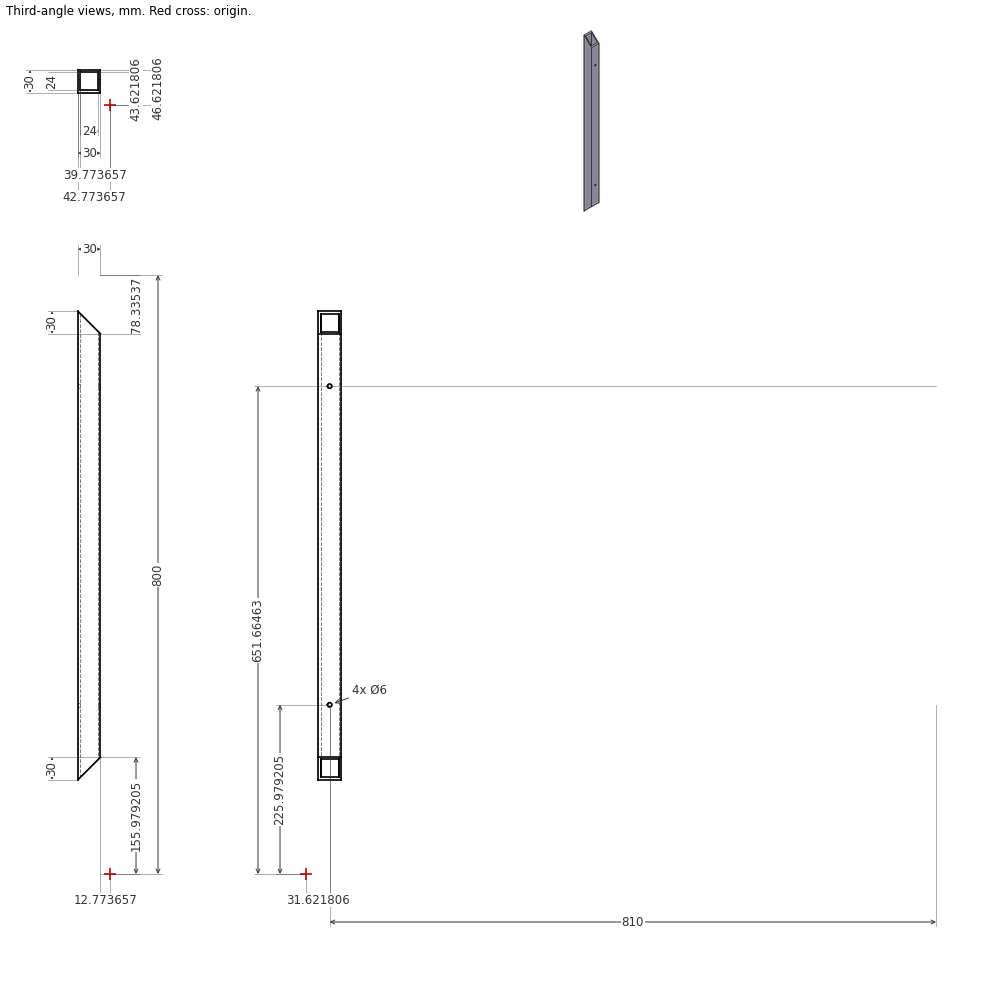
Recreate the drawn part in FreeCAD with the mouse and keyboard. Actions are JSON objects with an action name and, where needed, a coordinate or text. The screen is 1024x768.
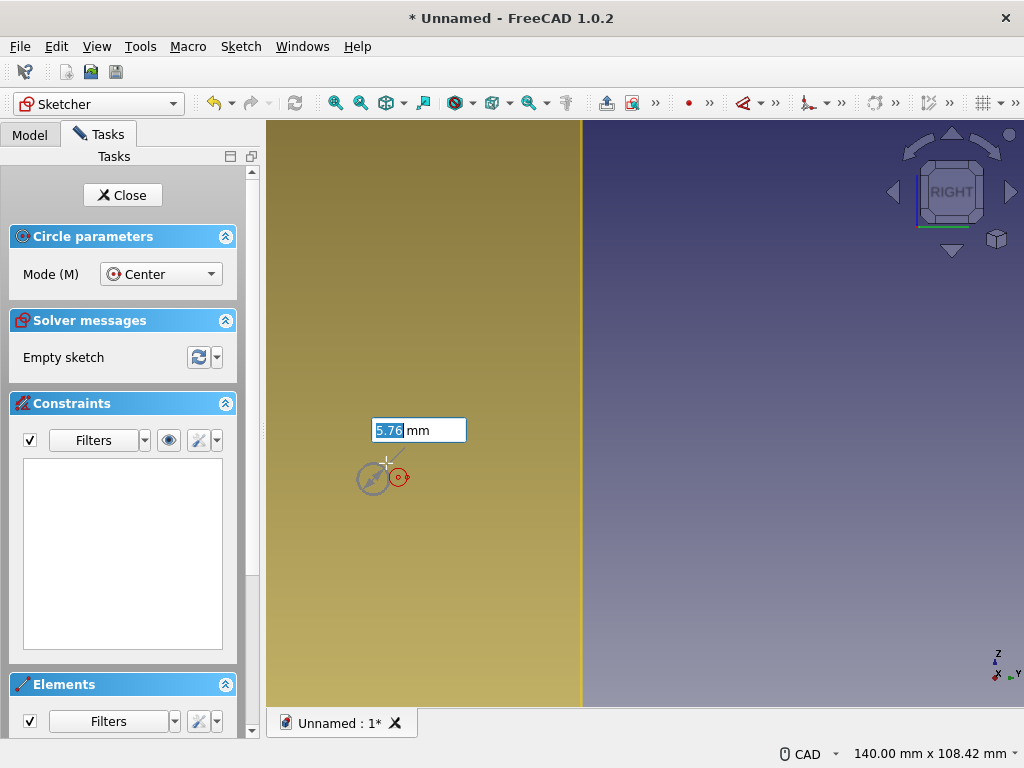
{"action": "left_click", "coordinate": [384, 454]}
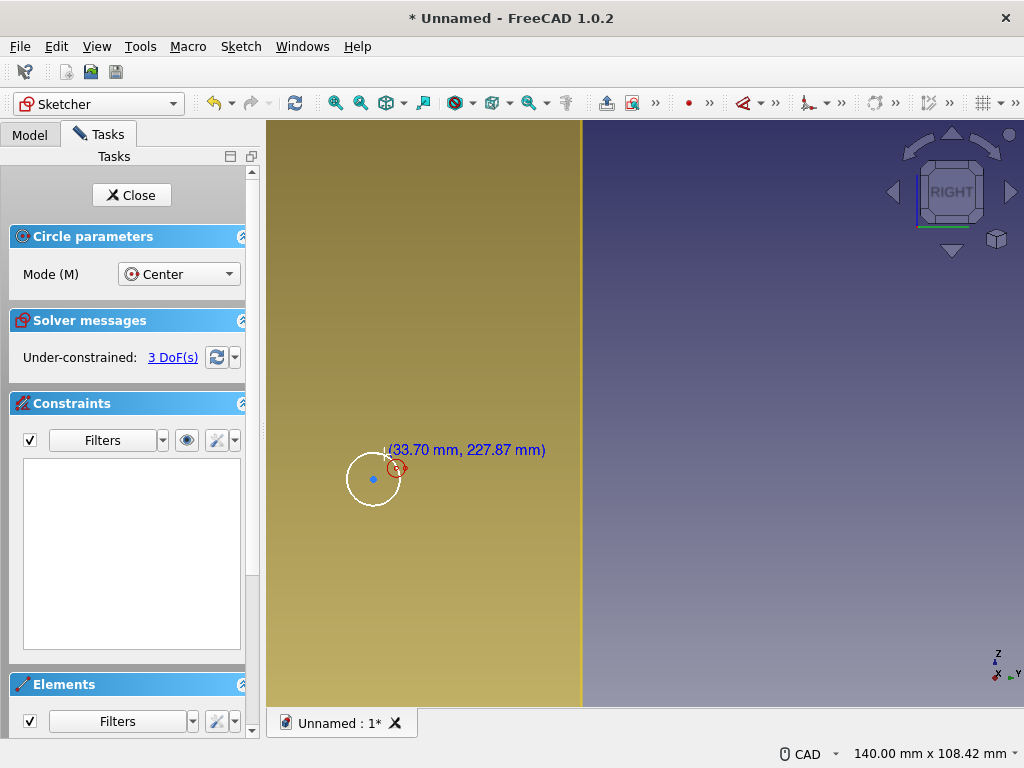
{"action": "scroll", "coordinate": [386, 463], "scroll_direction": "down", "scroll_amount": 12}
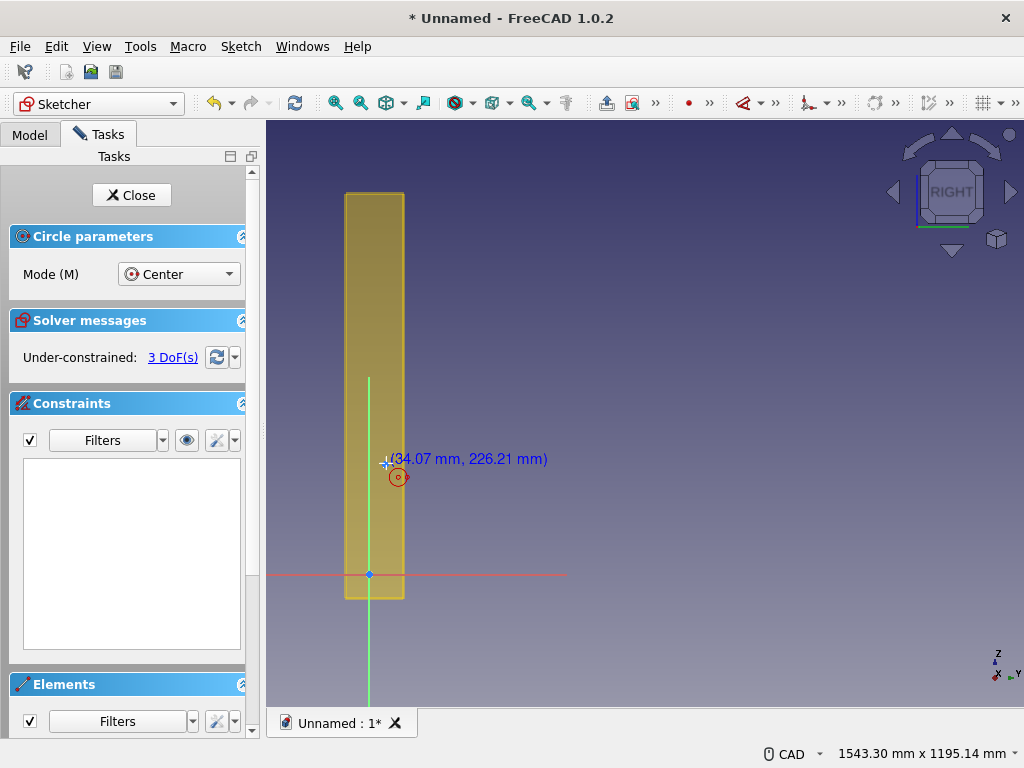
{"action": "scroll", "coordinate": [783, 464], "scroll_direction": "up", "scroll_amount": 14}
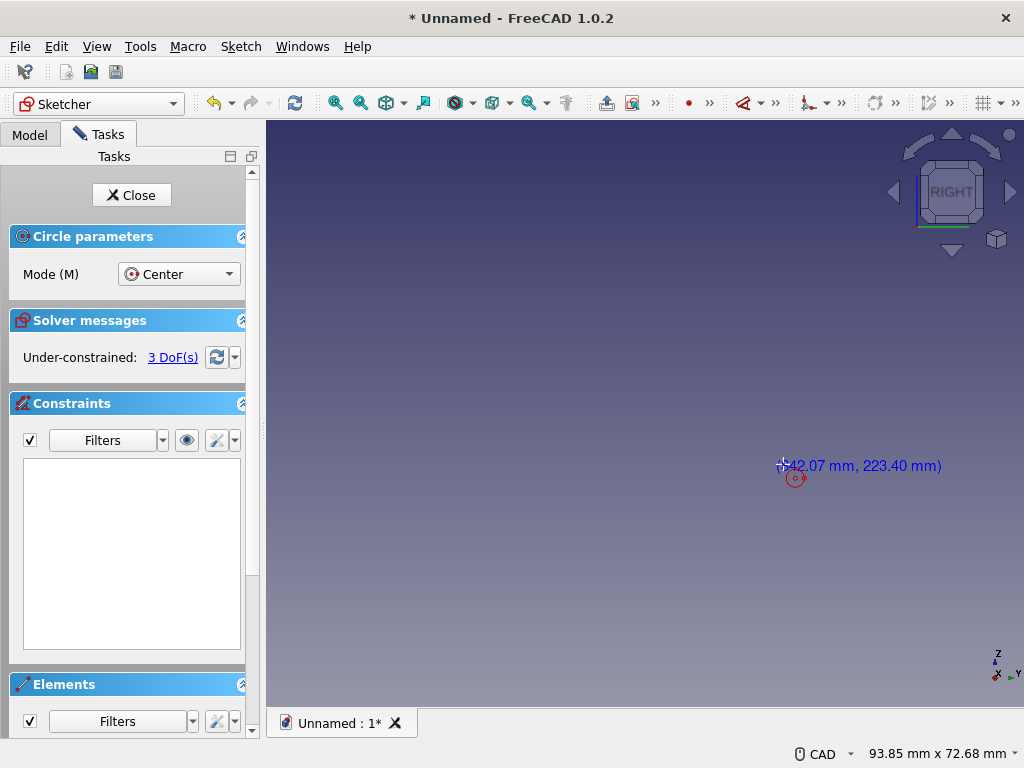
{"action": "scroll", "coordinate": [783, 464], "scroll_direction": "down", "scroll_amount": 14}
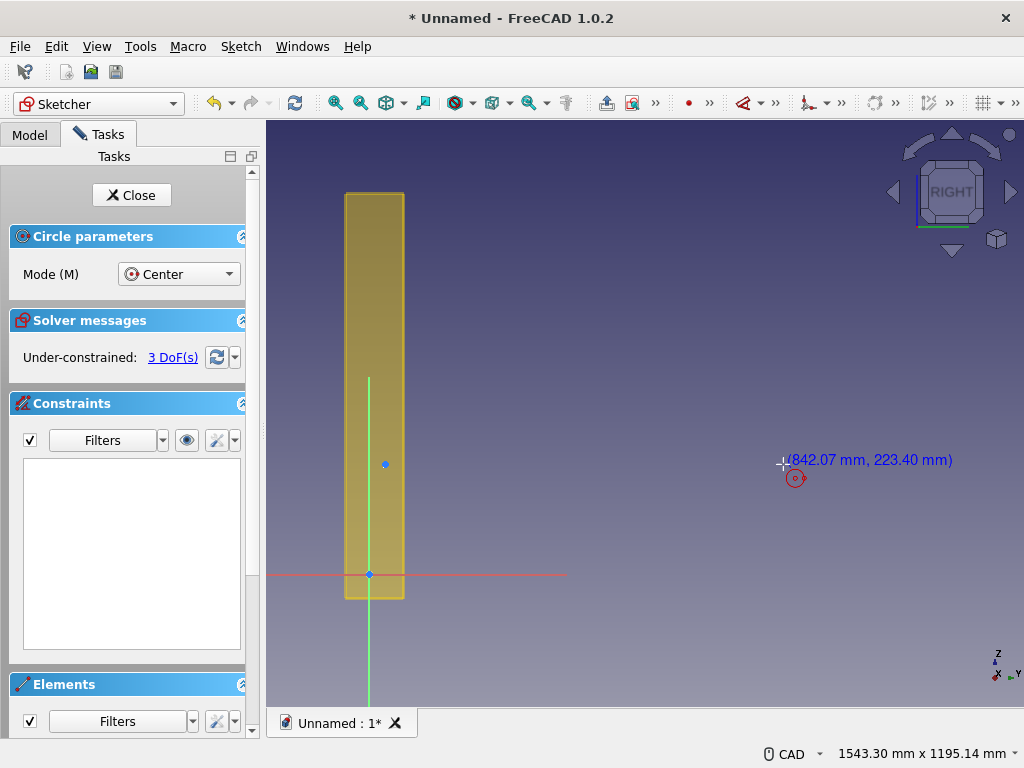
{"action": "left_click", "coordinate": [783, 464]}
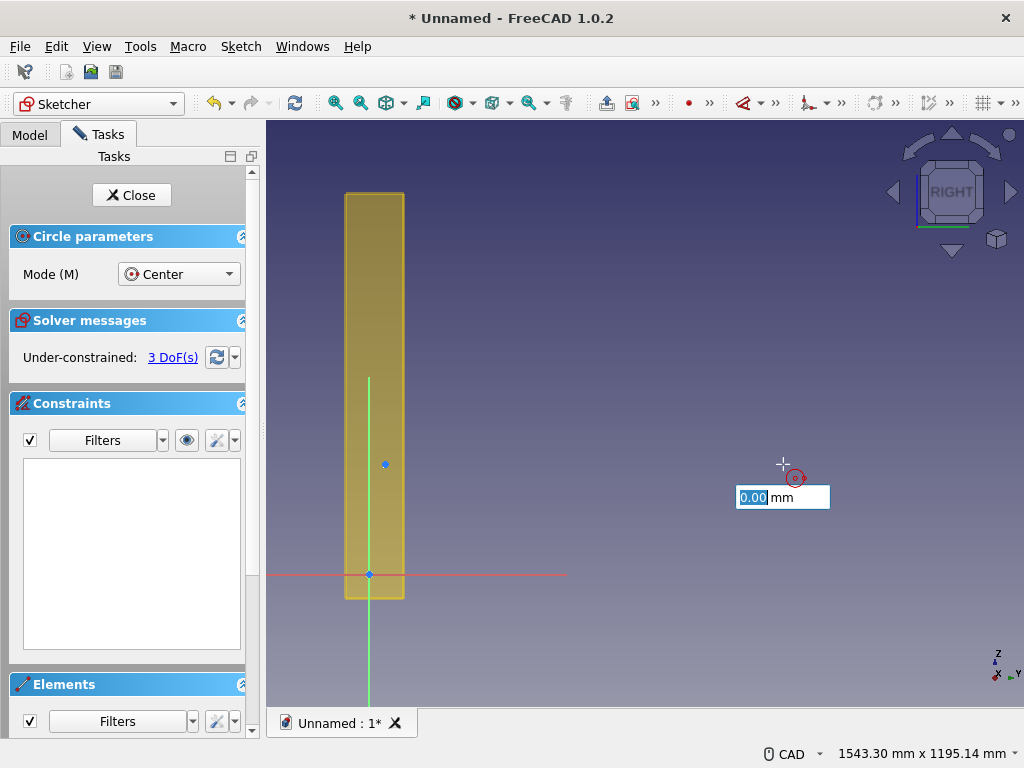
{"action": "scroll", "coordinate": [784, 463], "scroll_direction": "up", "scroll_amount": 12}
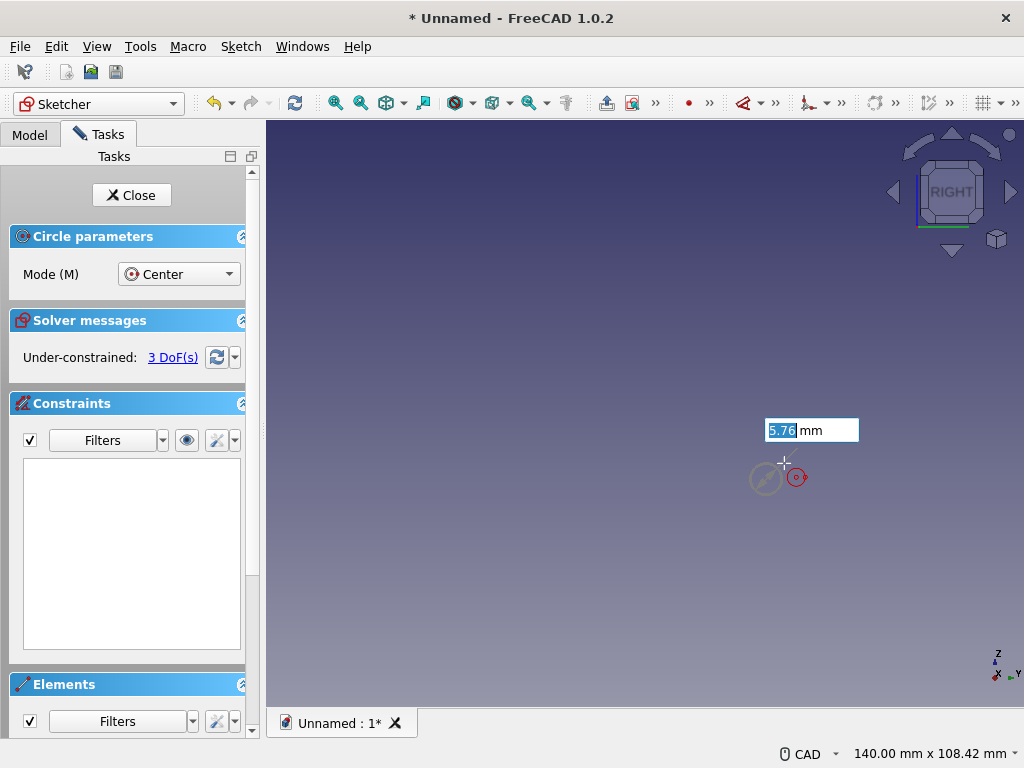
{"action": "left_click", "coordinate": [775, 454]}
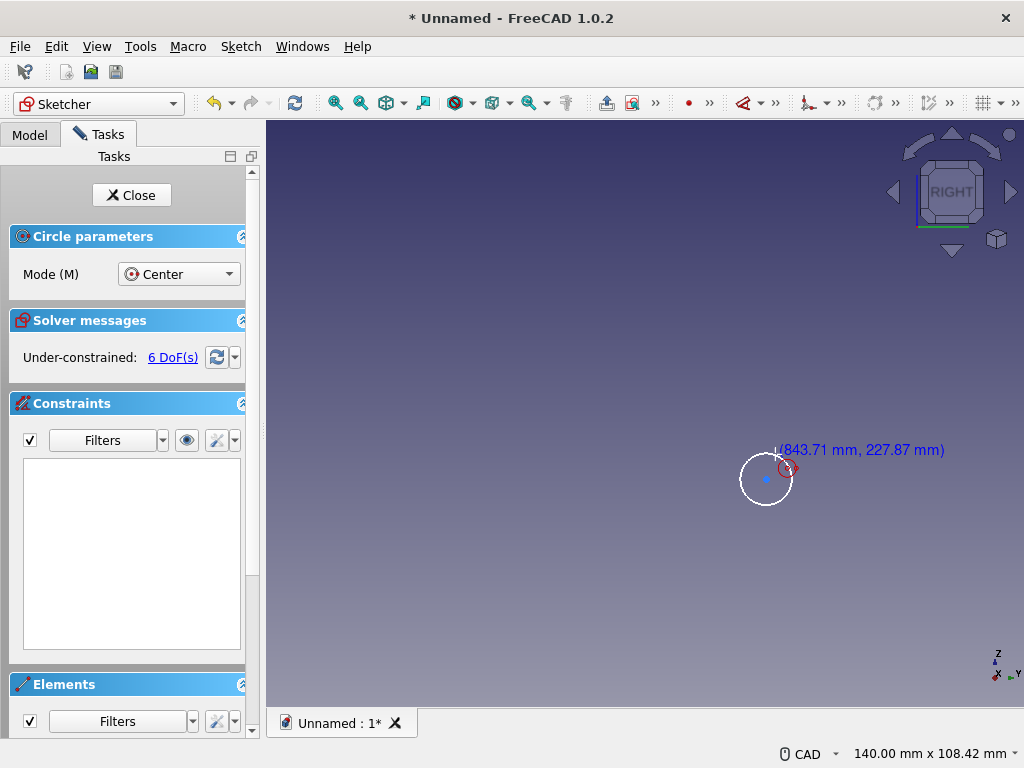
{"action": "scroll", "coordinate": [784, 463], "scroll_direction": "down", "scroll_amount": 12}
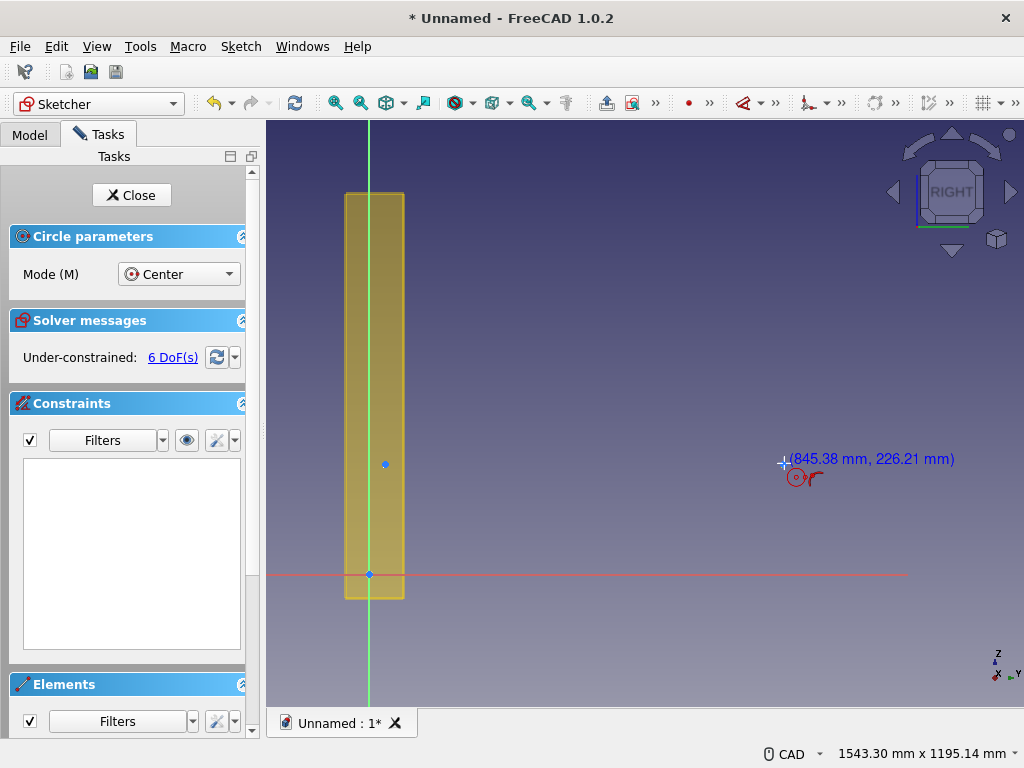
{"action": "scroll", "coordinate": [783, 255], "scroll_direction": "up", "scroll_amount": 14}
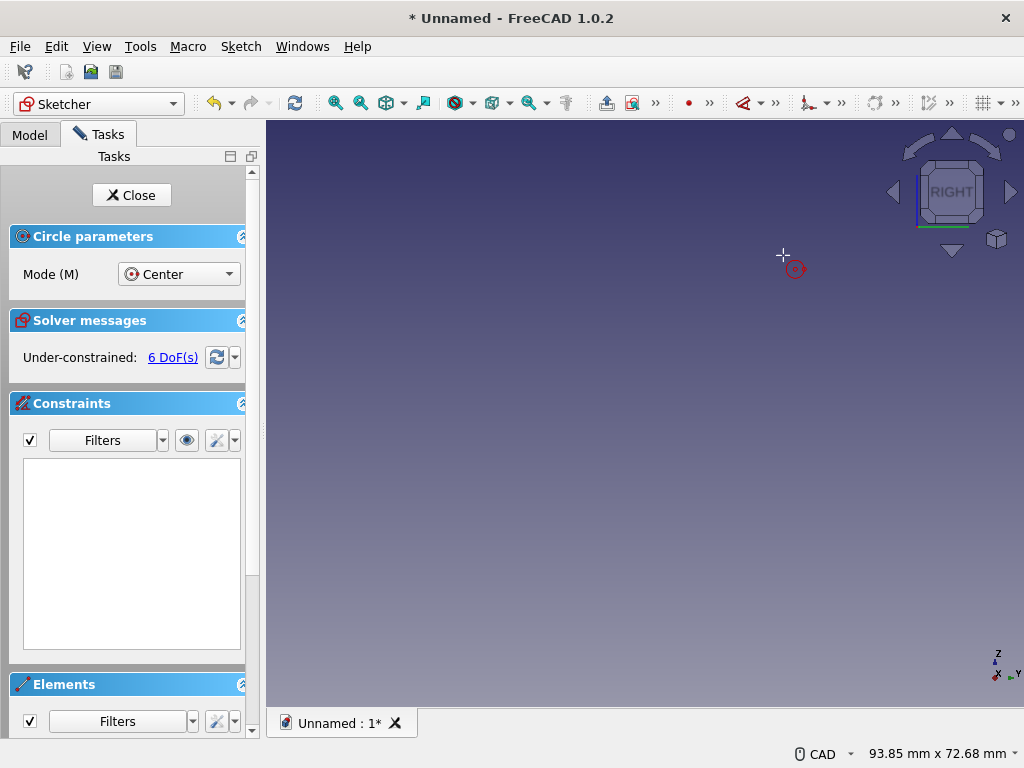
{"action": "scroll", "coordinate": [783, 255], "scroll_direction": "down", "scroll_amount": 14}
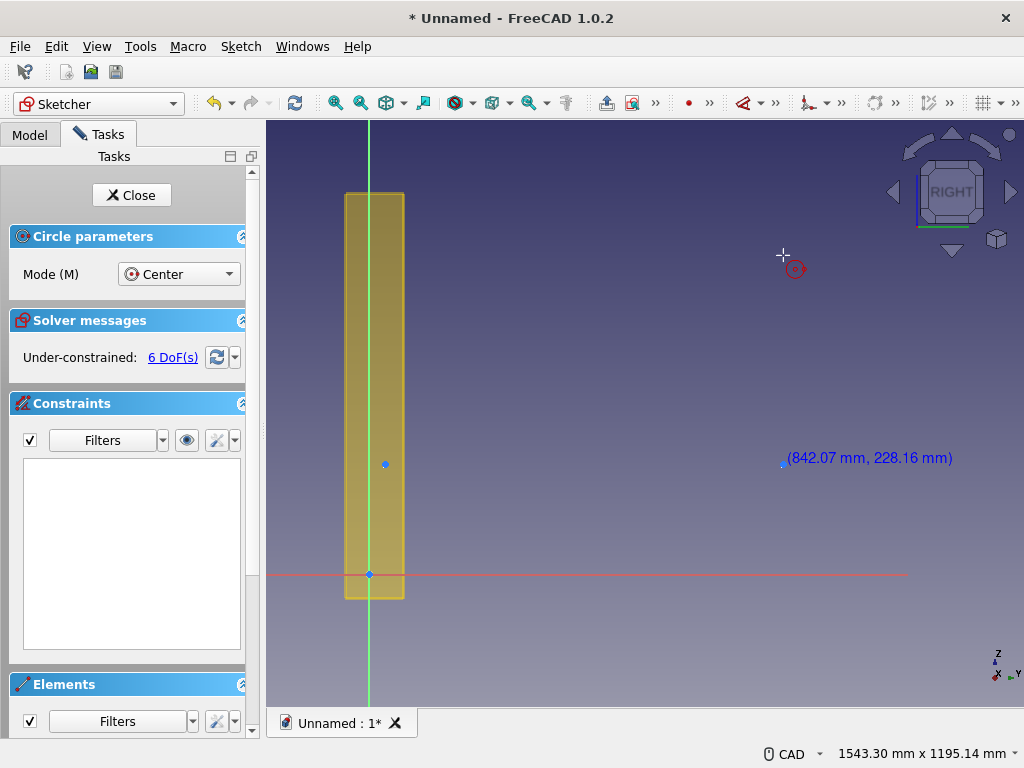
{"action": "left_click", "coordinate": [783, 255]}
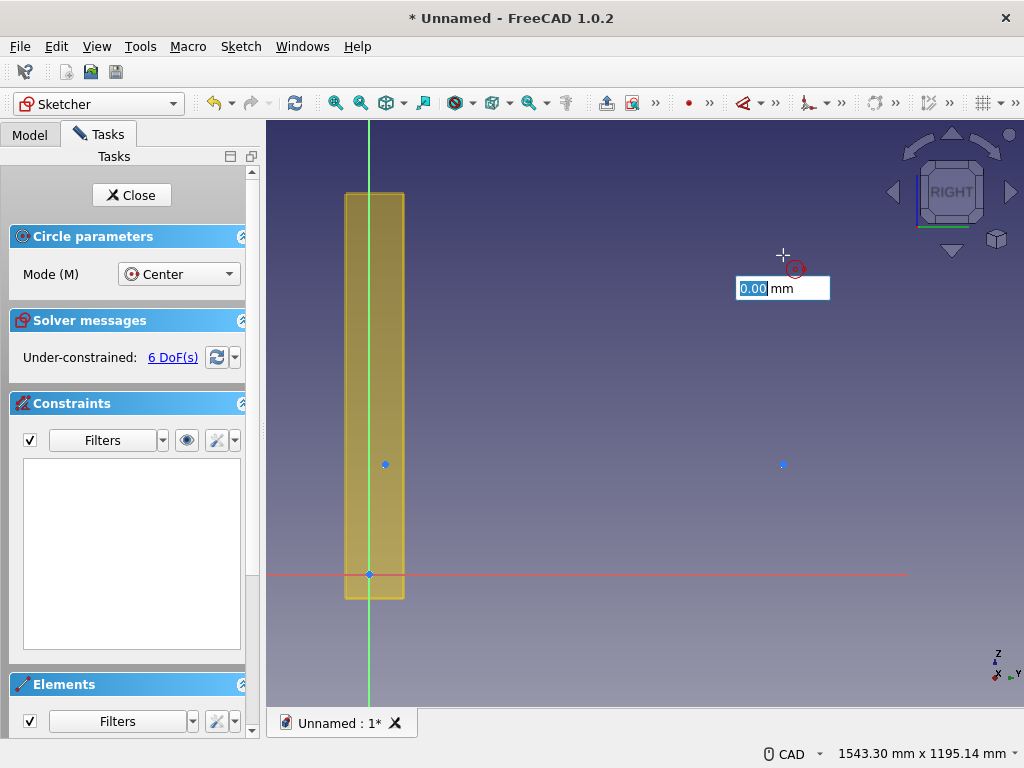
{"action": "scroll", "coordinate": [784, 254], "scroll_direction": "up", "scroll_amount": 12}